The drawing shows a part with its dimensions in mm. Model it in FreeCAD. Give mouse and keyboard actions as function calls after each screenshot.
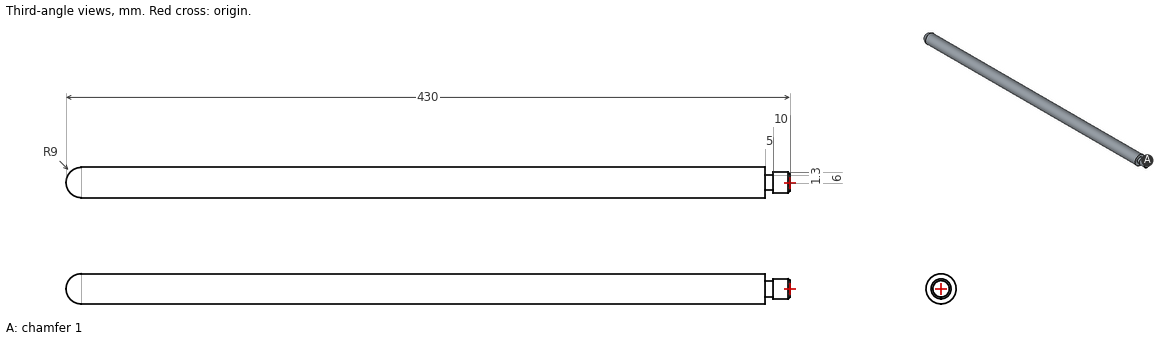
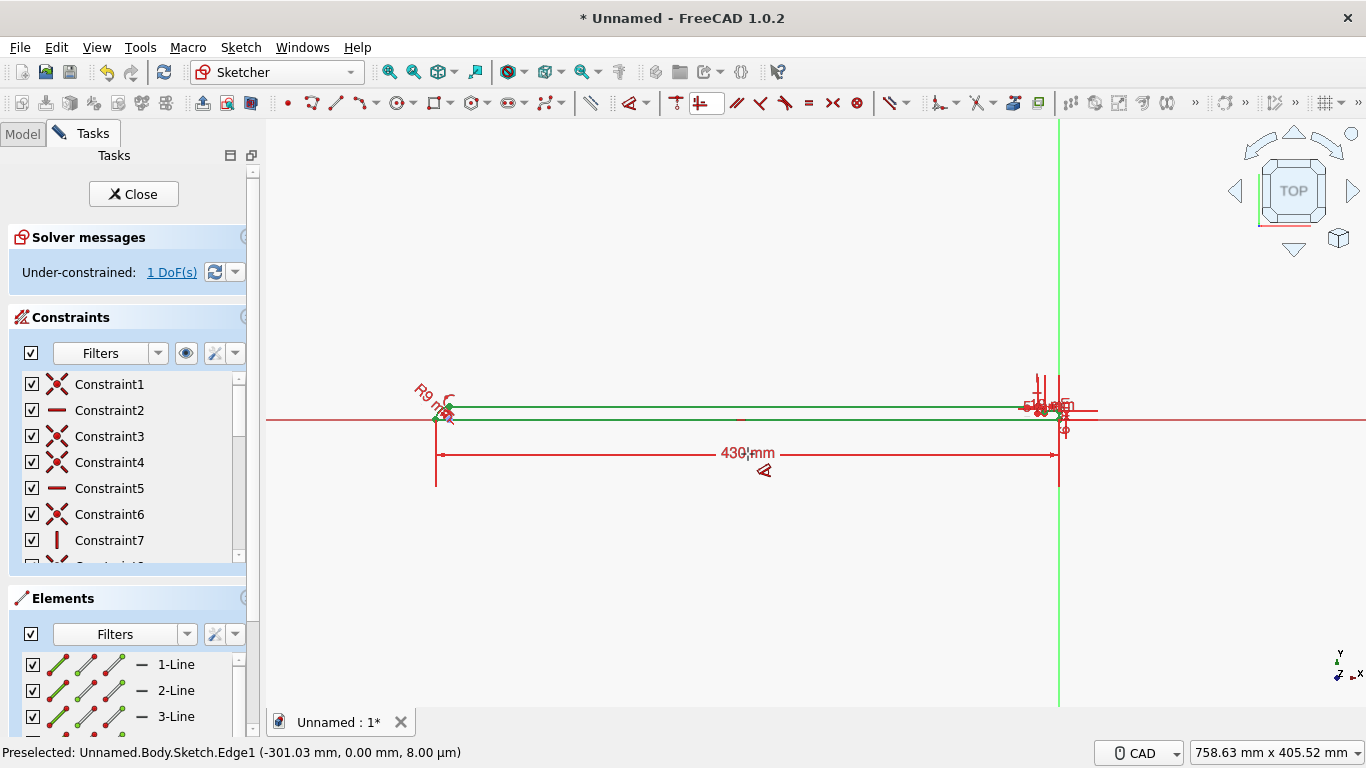
scroll(1045, 412, up, 16)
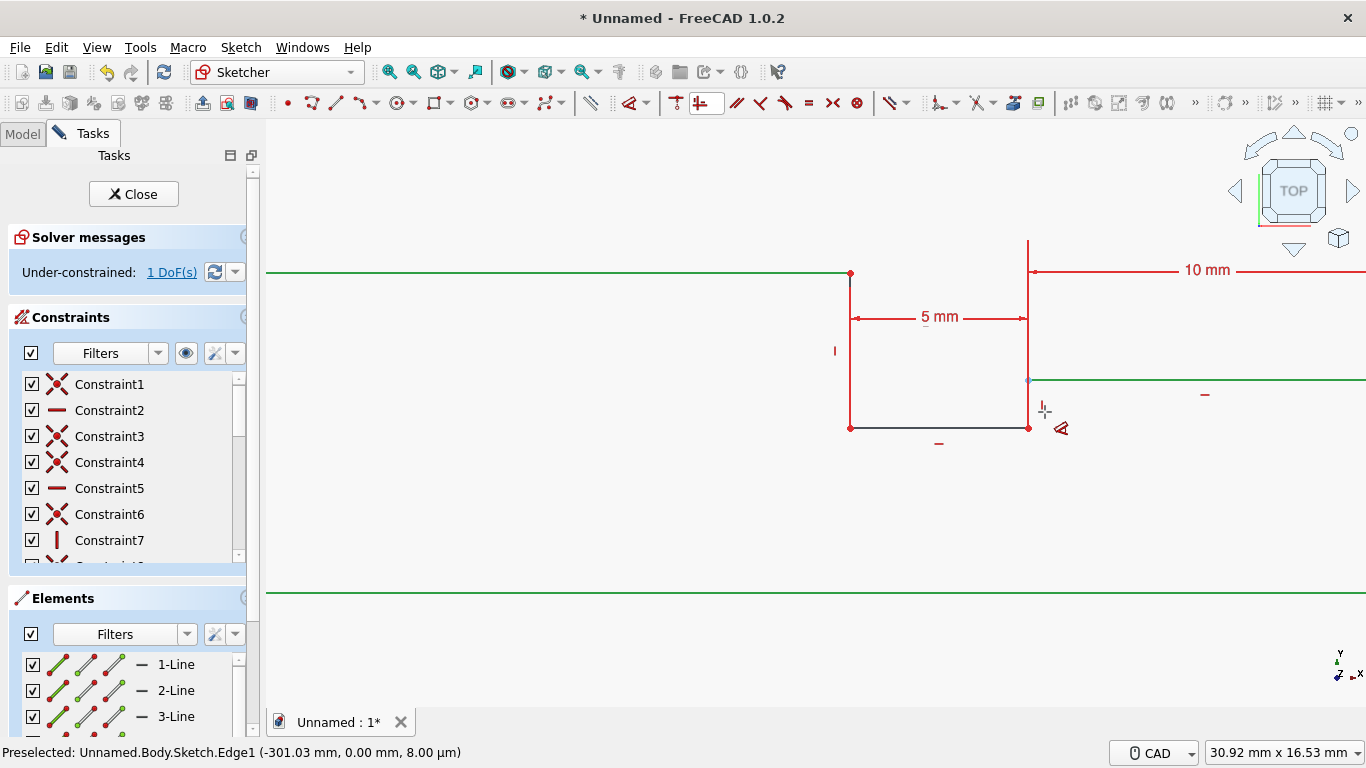
click(1028, 404)
click(1062, 404)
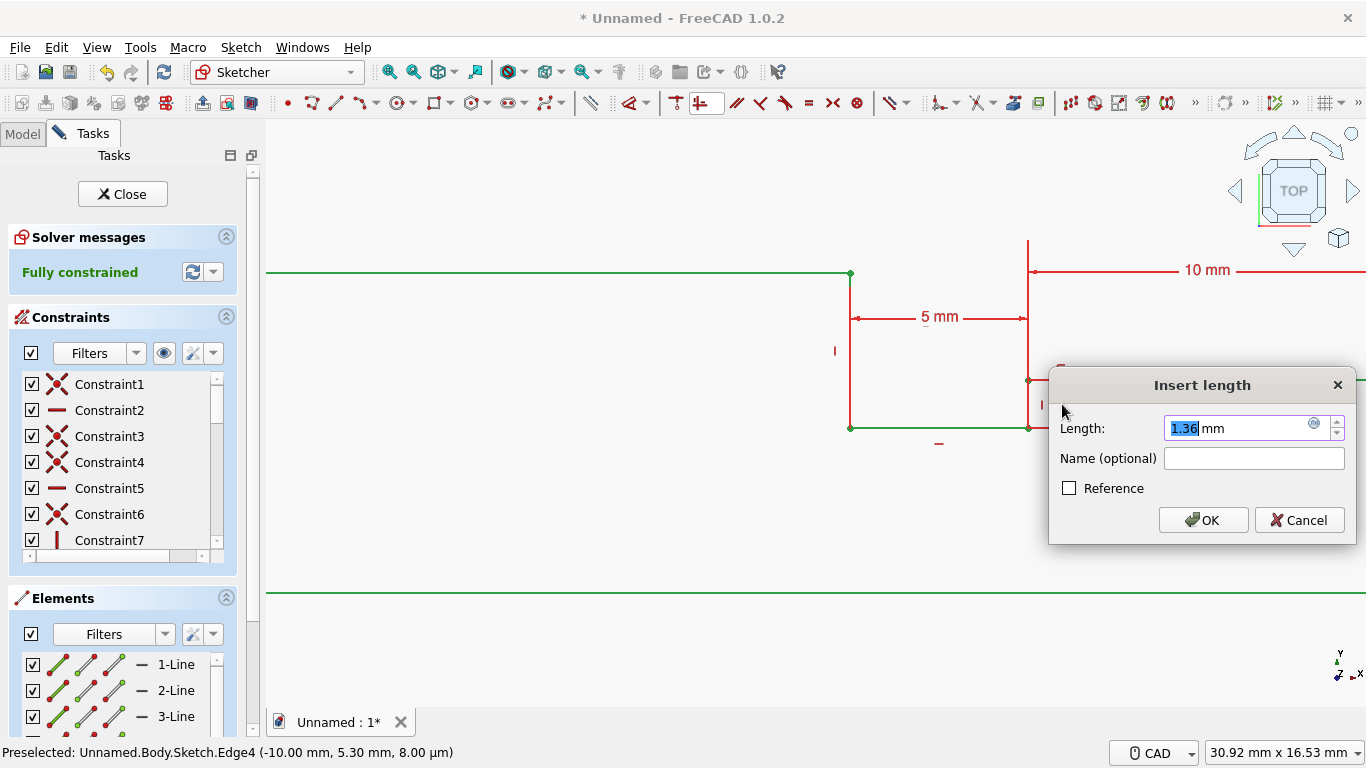
text(1.3)
key(Return)
key(Escape)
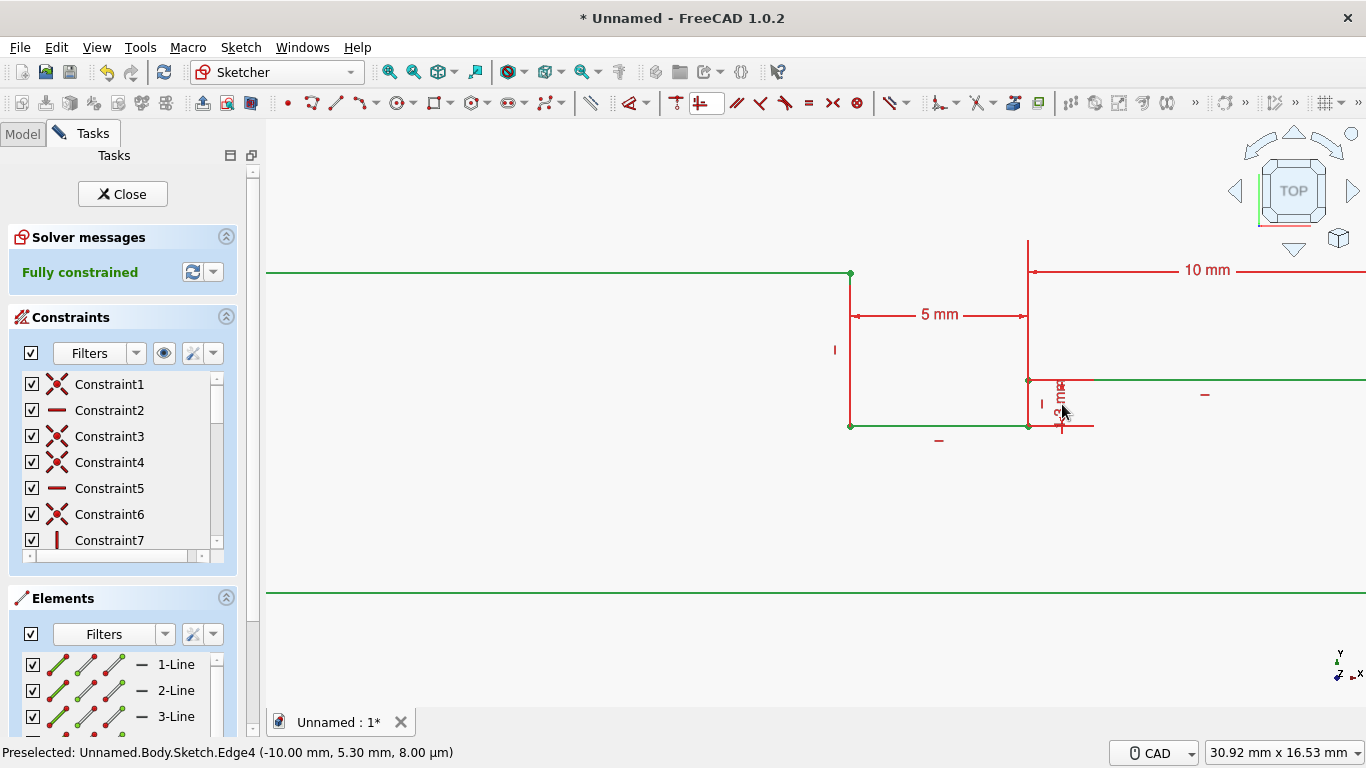
click(123, 194)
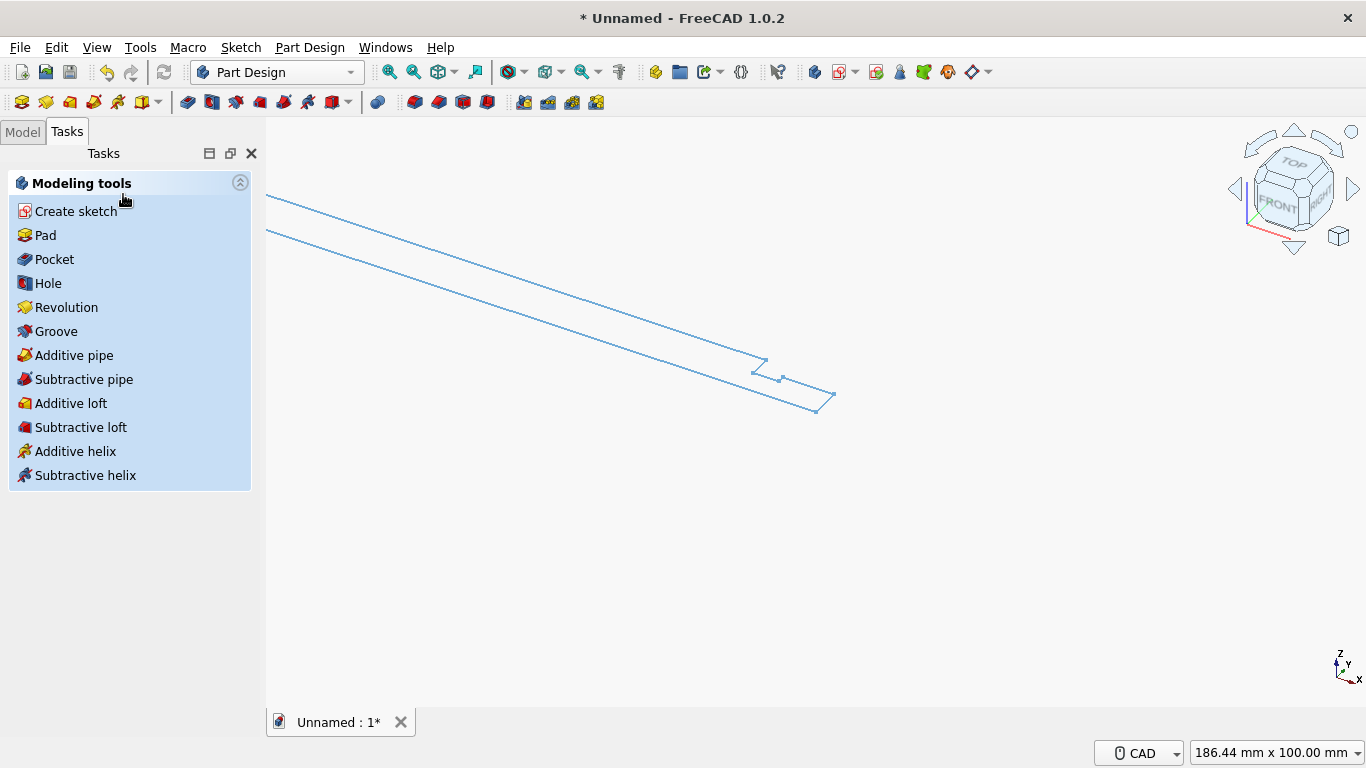
click(46, 102)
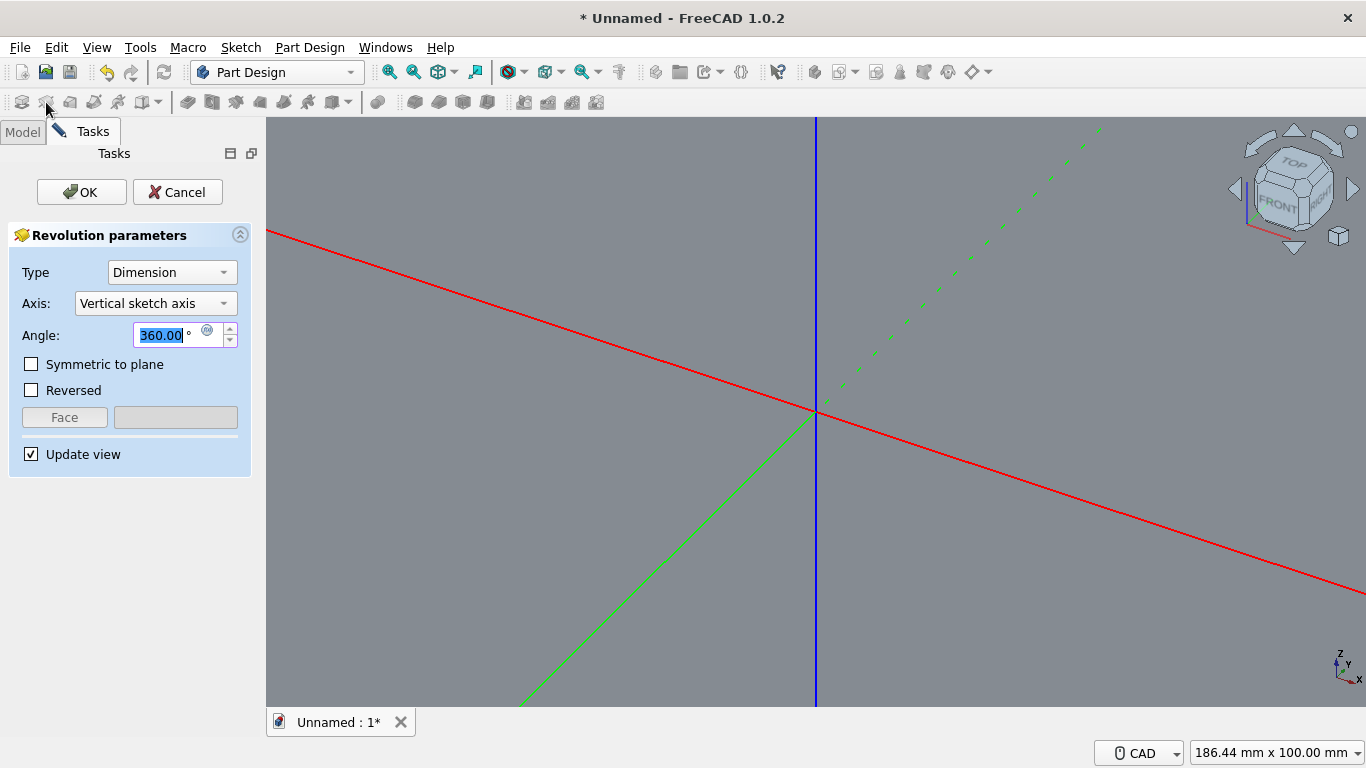
click(156, 304)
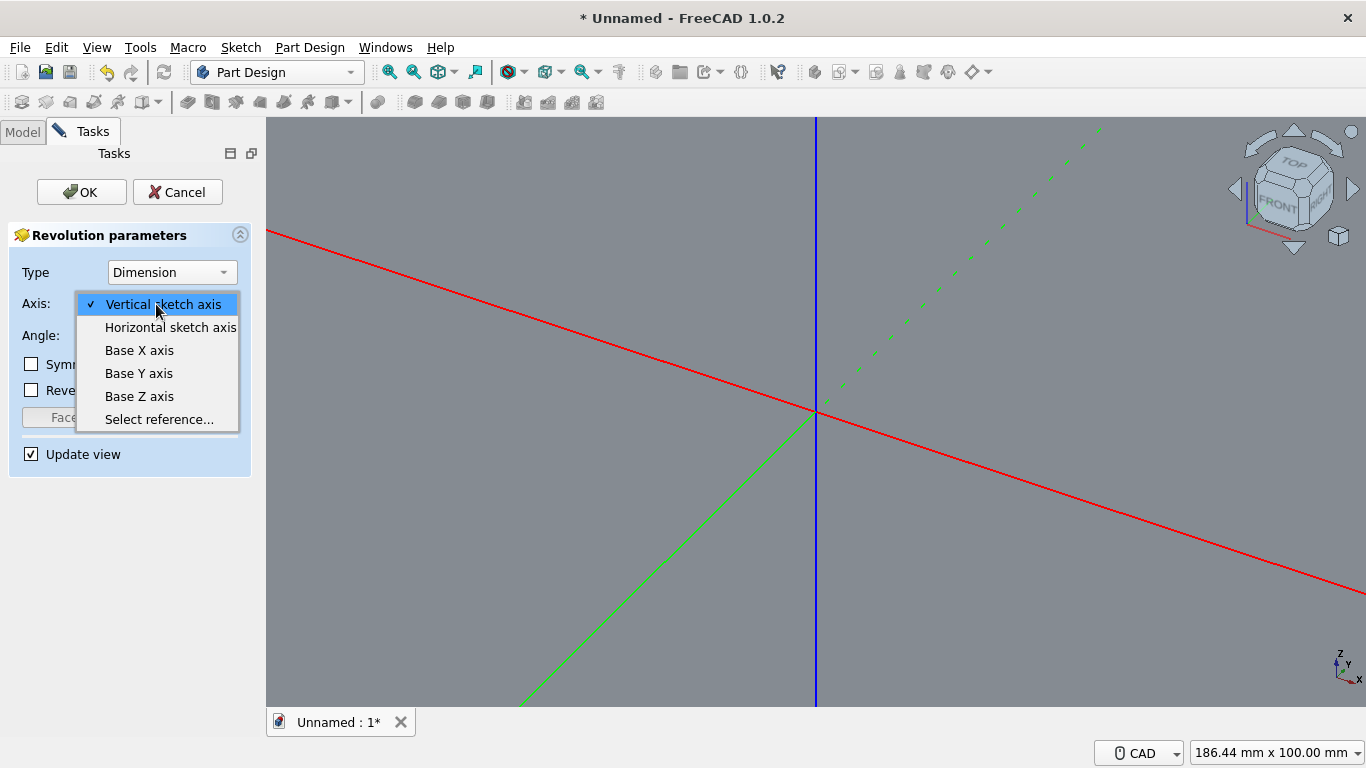
click(156, 328)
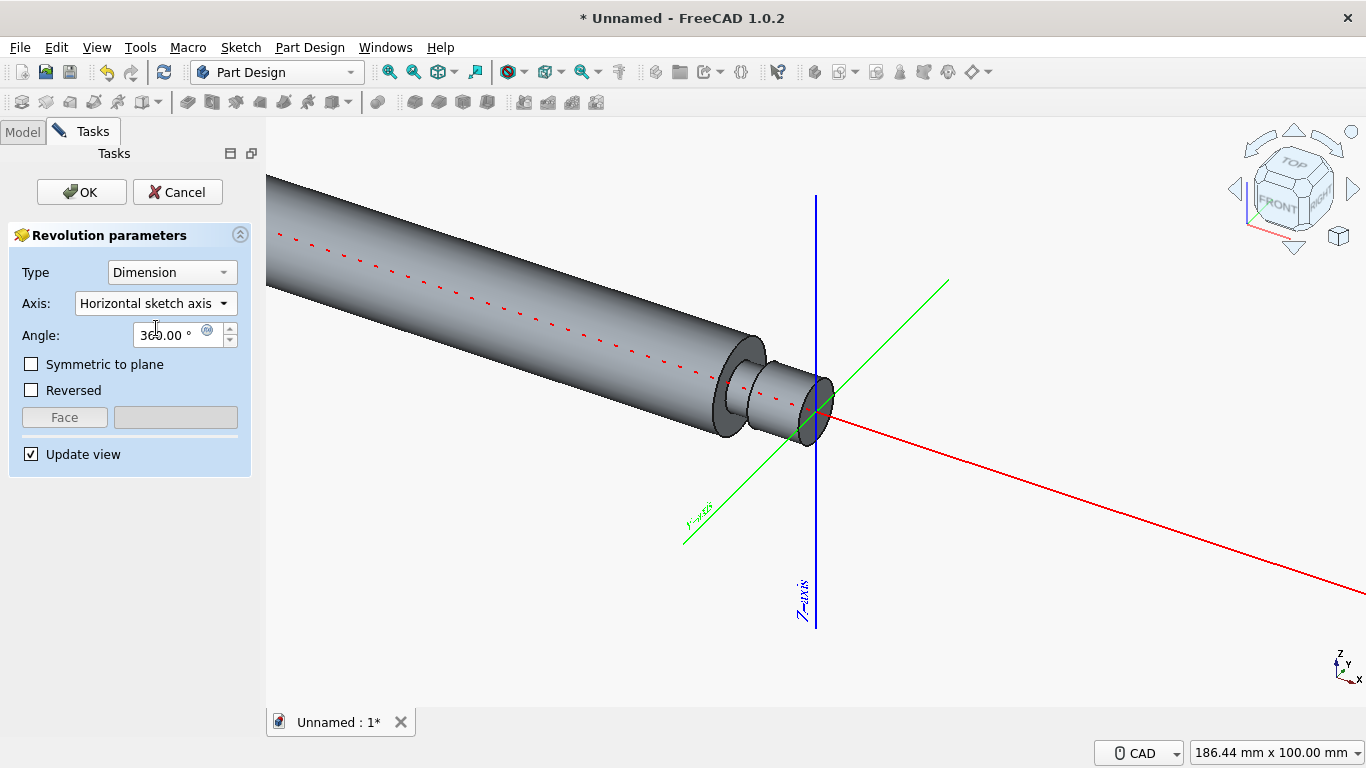
click(82, 192)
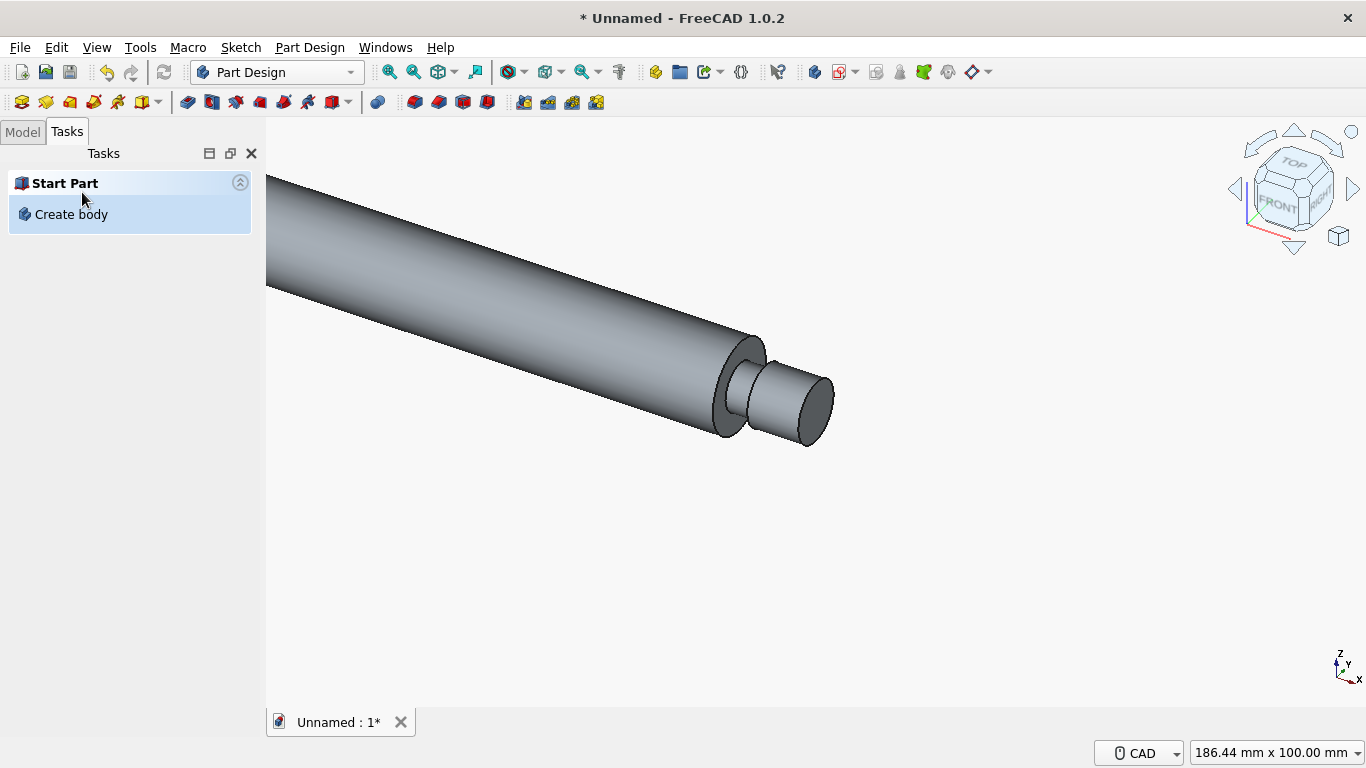
click(390, 72)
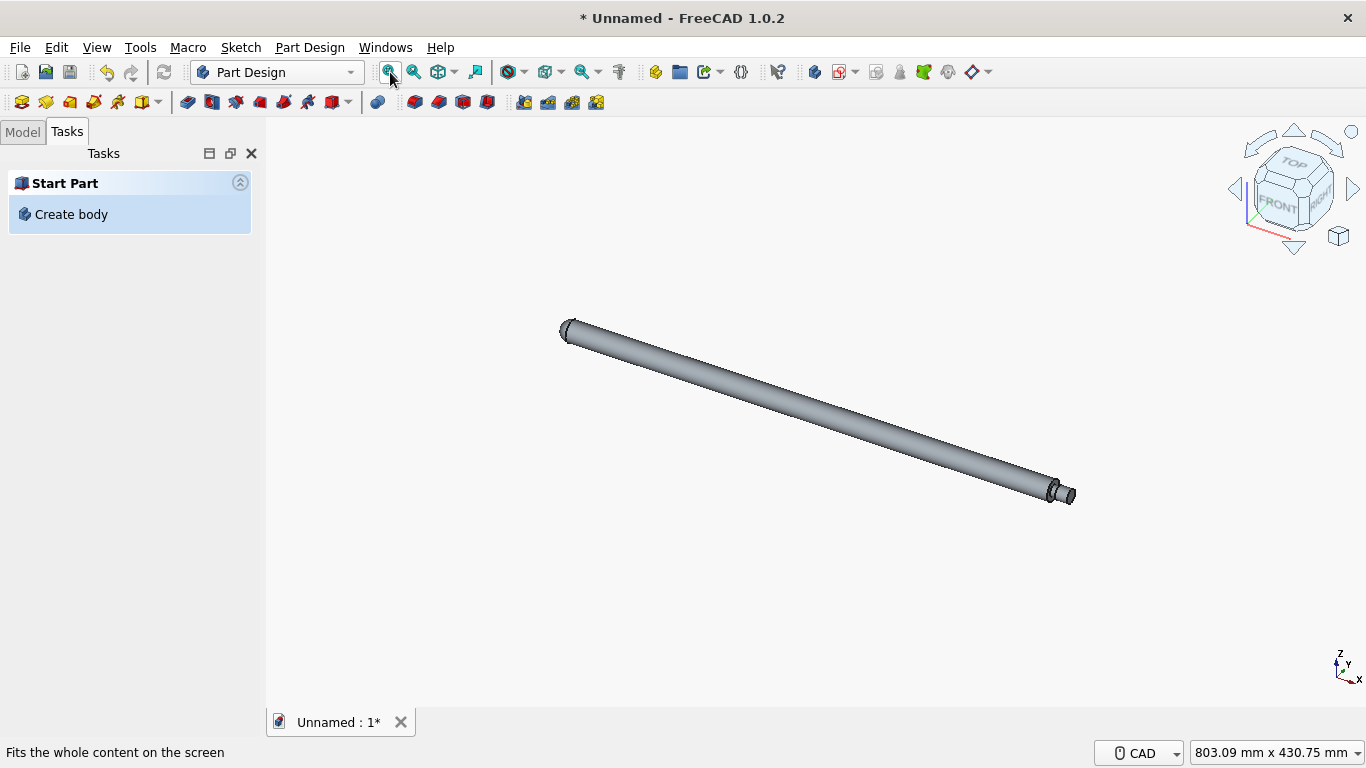
click(1067, 500)